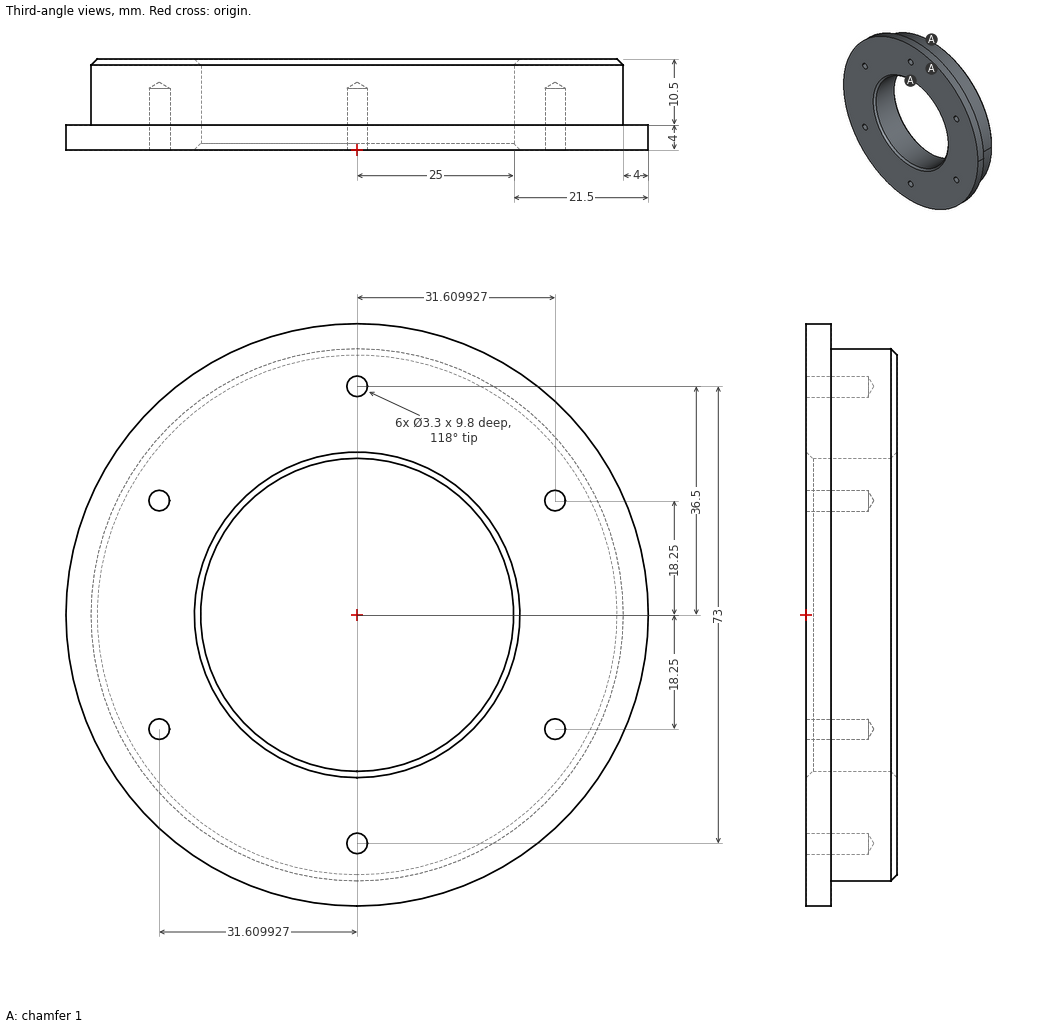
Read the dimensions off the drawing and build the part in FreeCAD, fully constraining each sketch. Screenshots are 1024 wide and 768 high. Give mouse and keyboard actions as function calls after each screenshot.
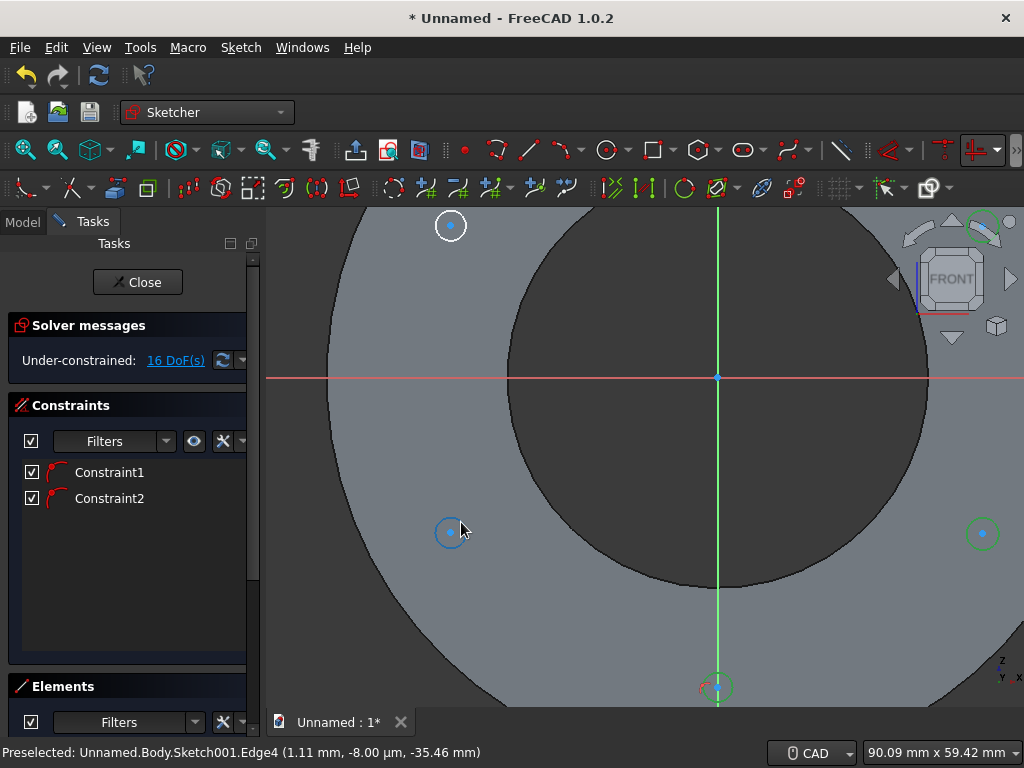
click(462, 522)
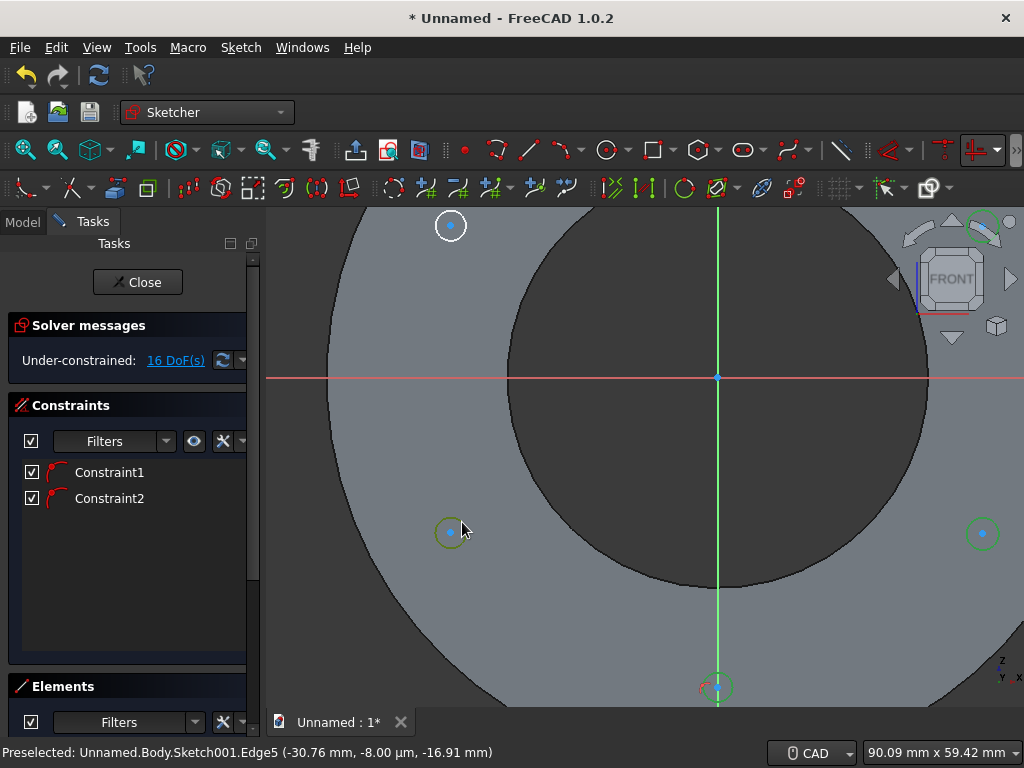
click(440, 236)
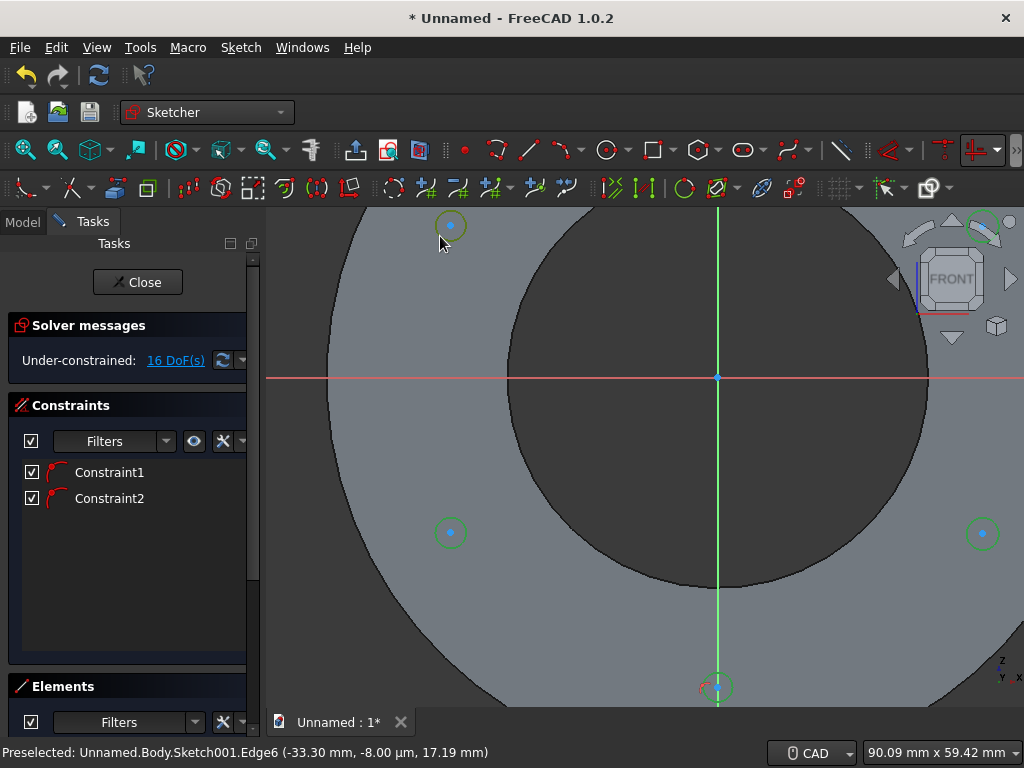
key(e)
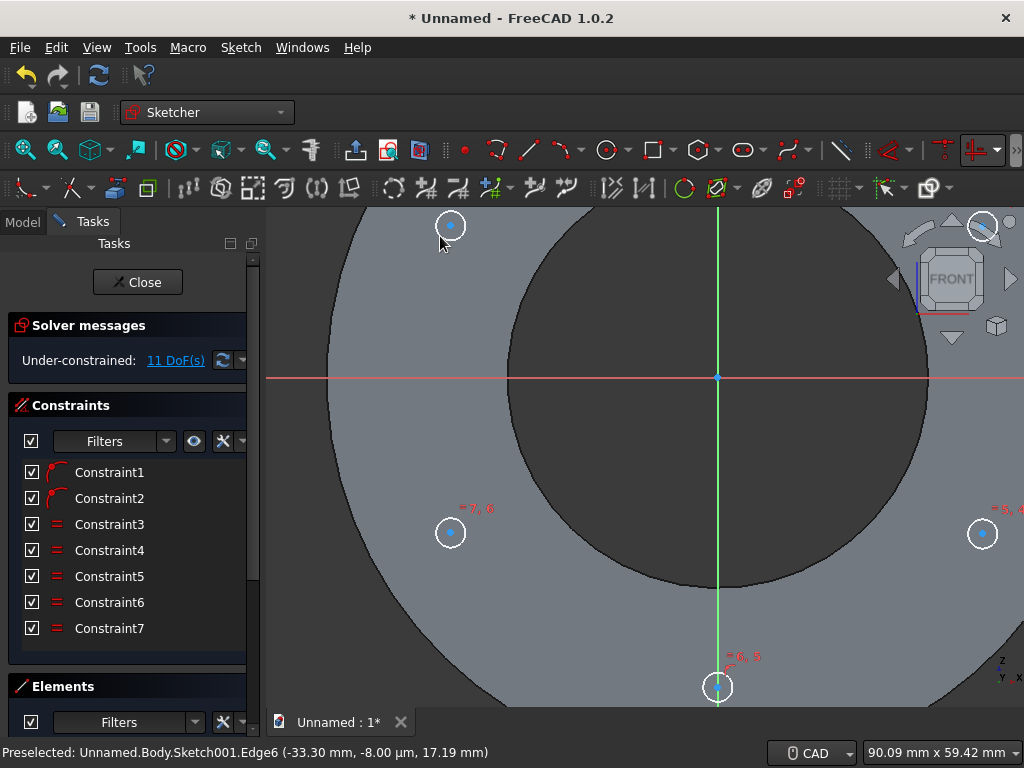
scroll(461, 522, down, 4)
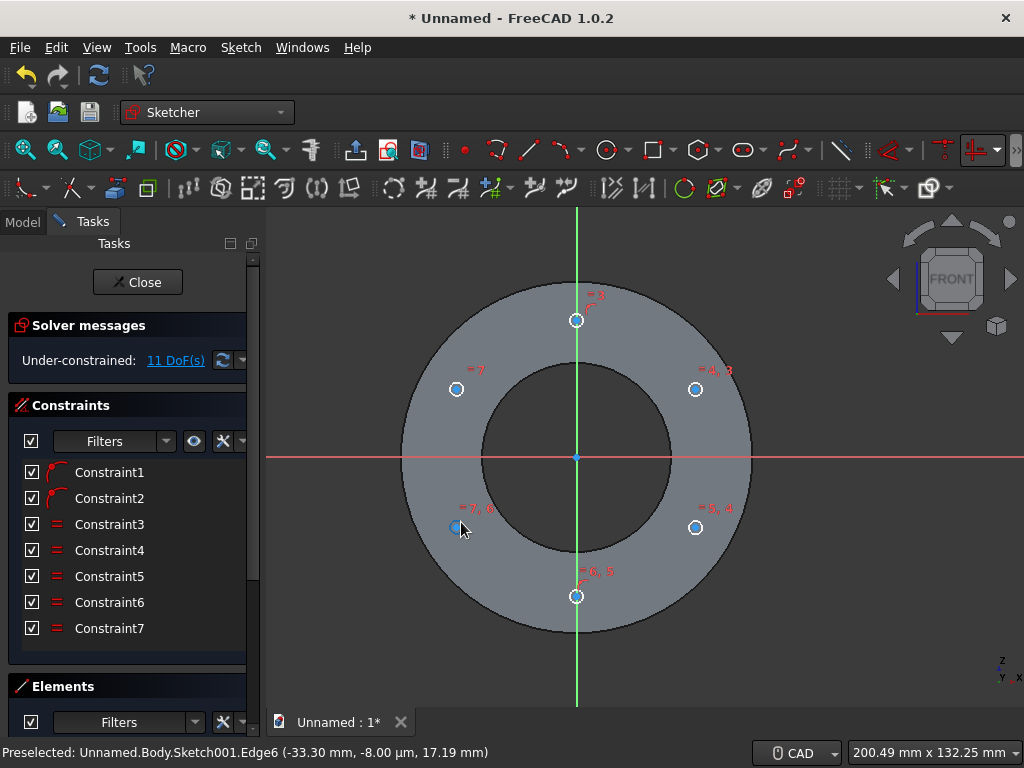
click(696, 389)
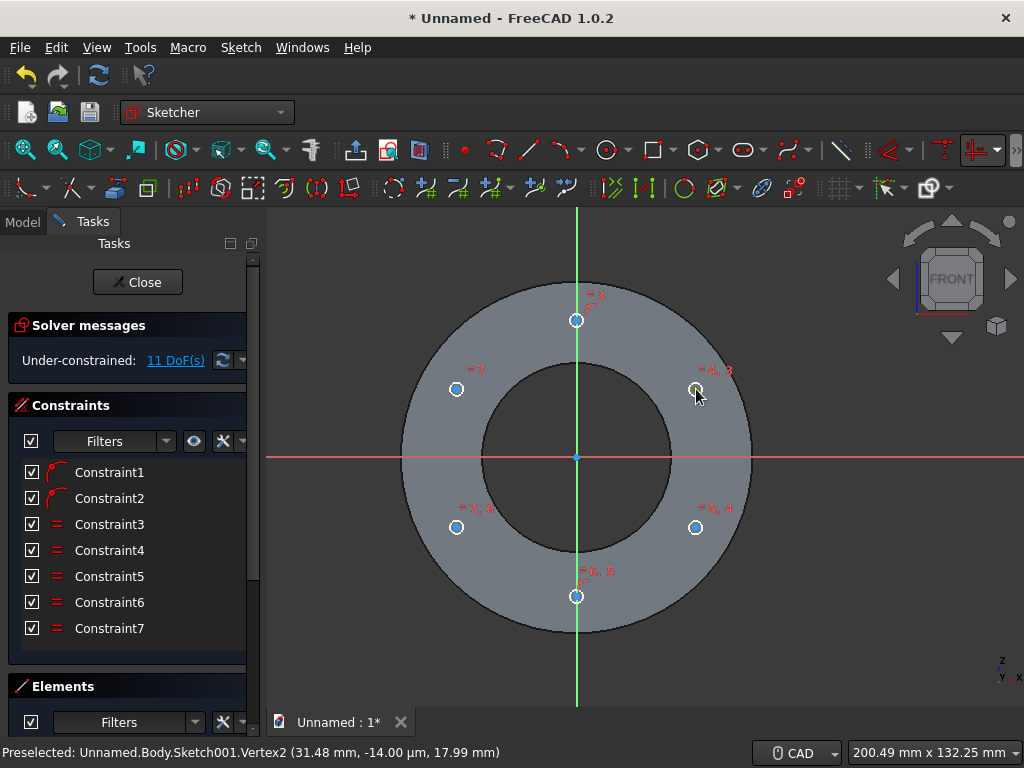
click(696, 528)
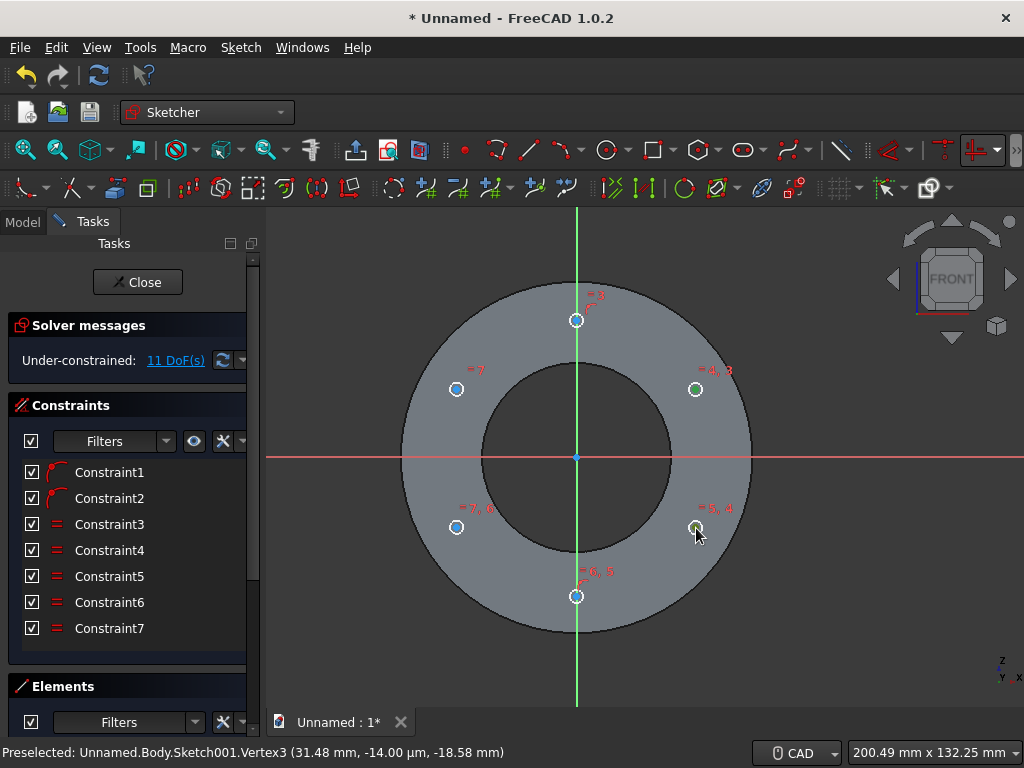
key(v)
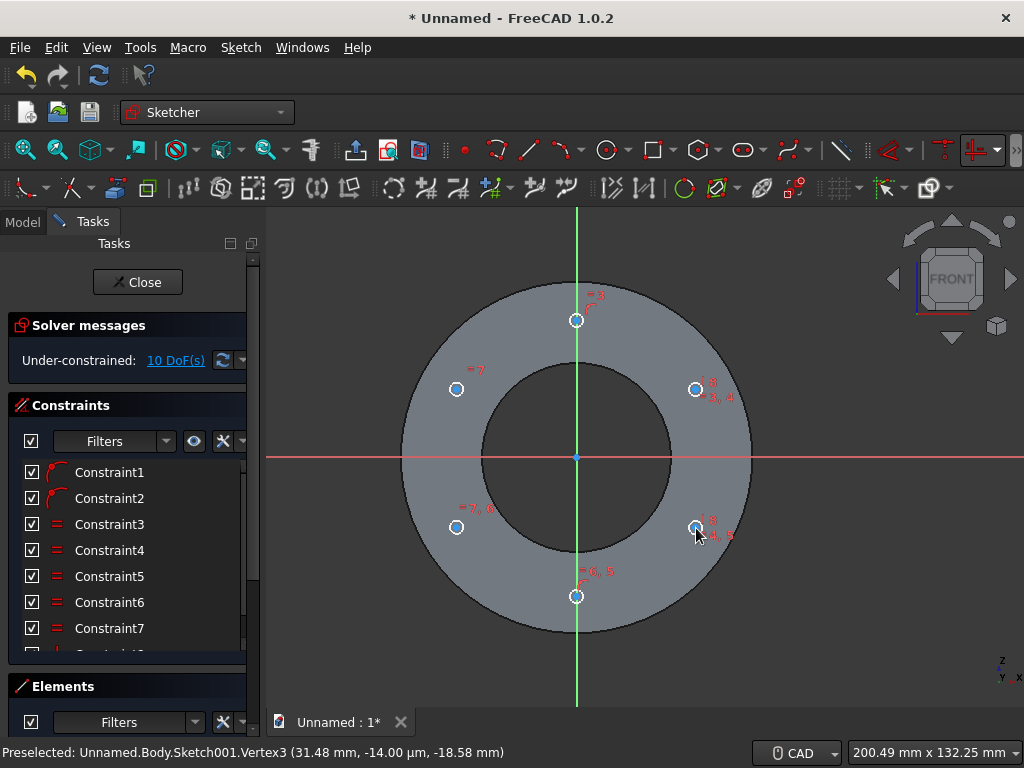
click(696, 528)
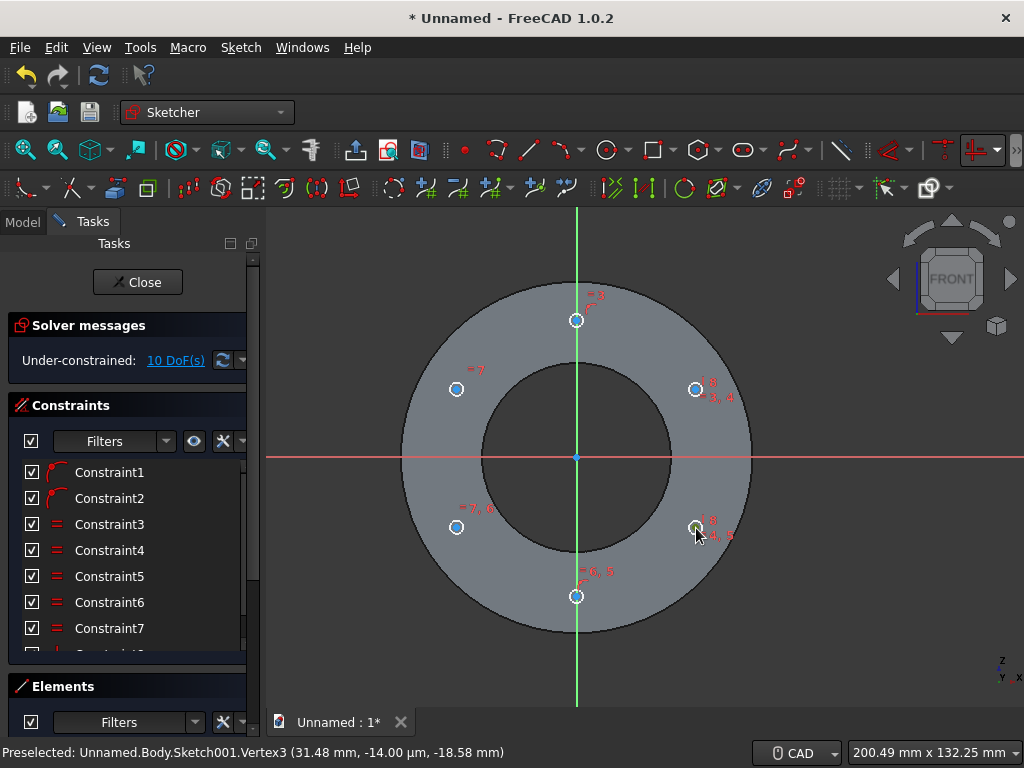
click(457, 527)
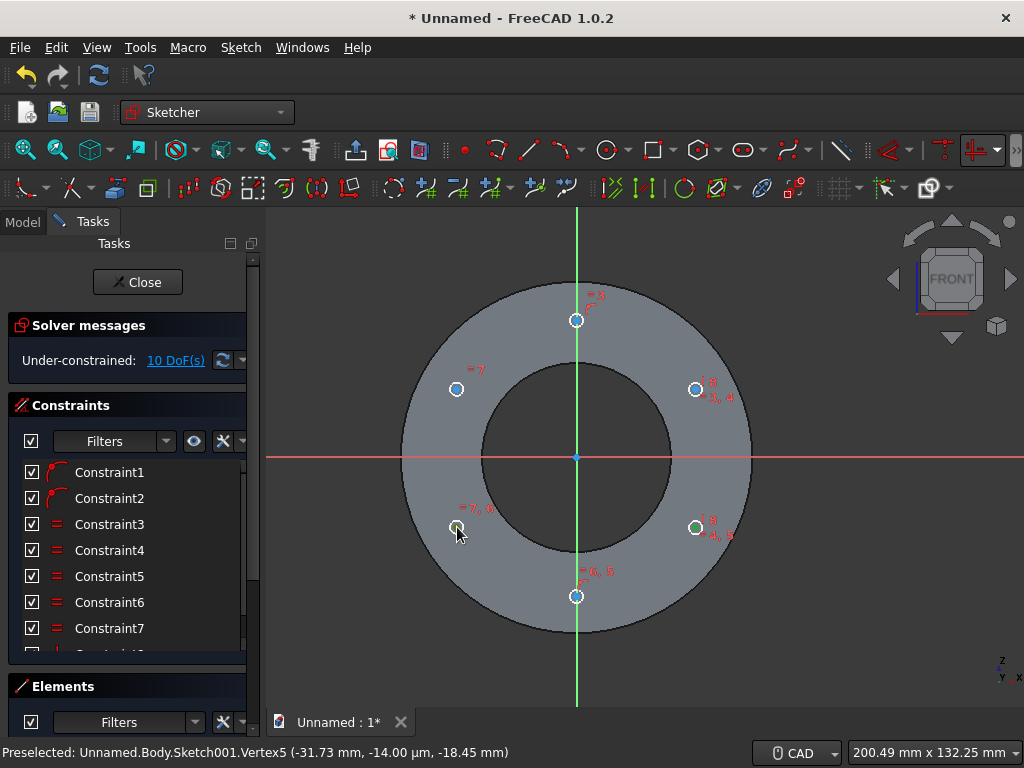
key(h)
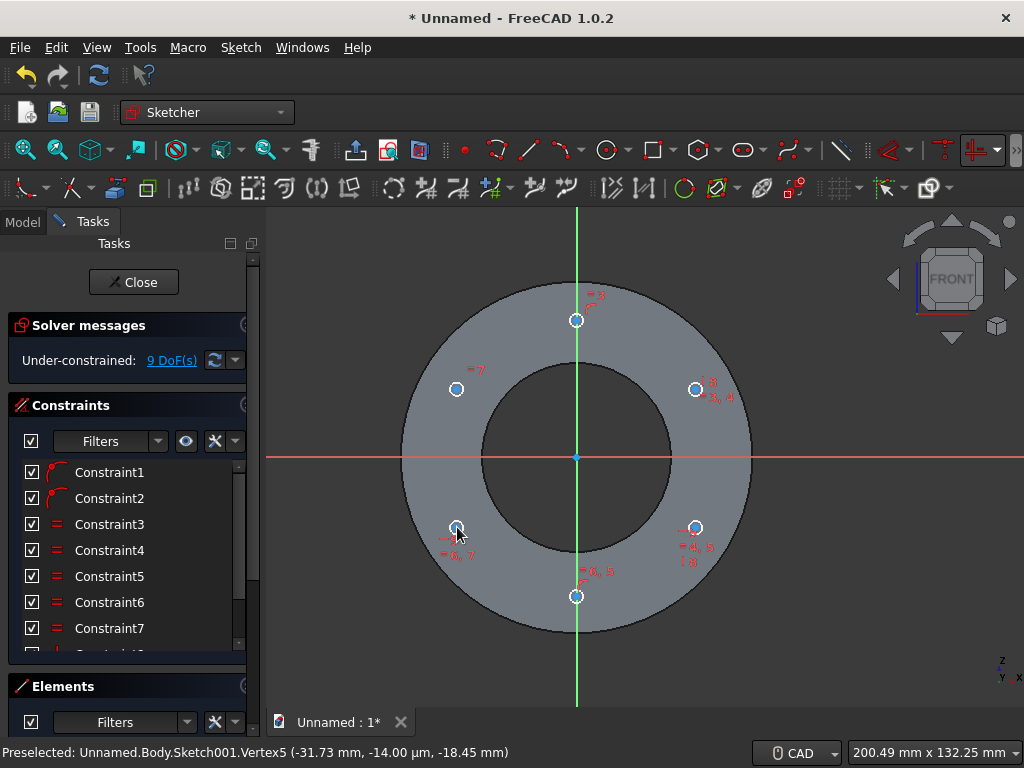
click(457, 528)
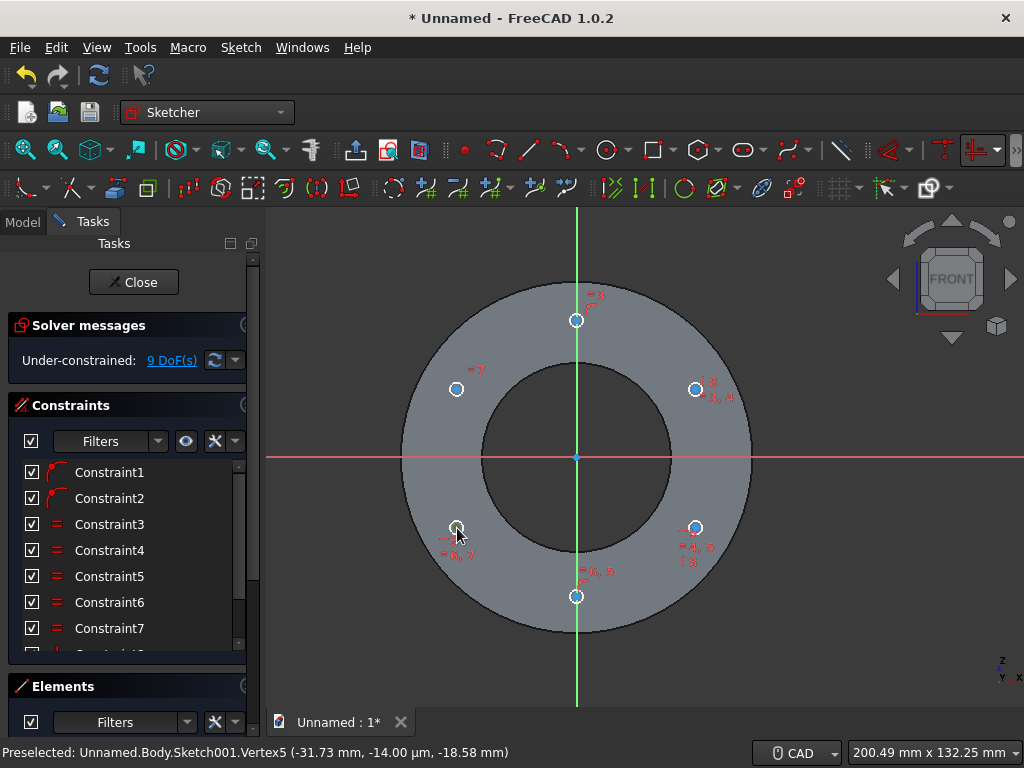
click(457, 389)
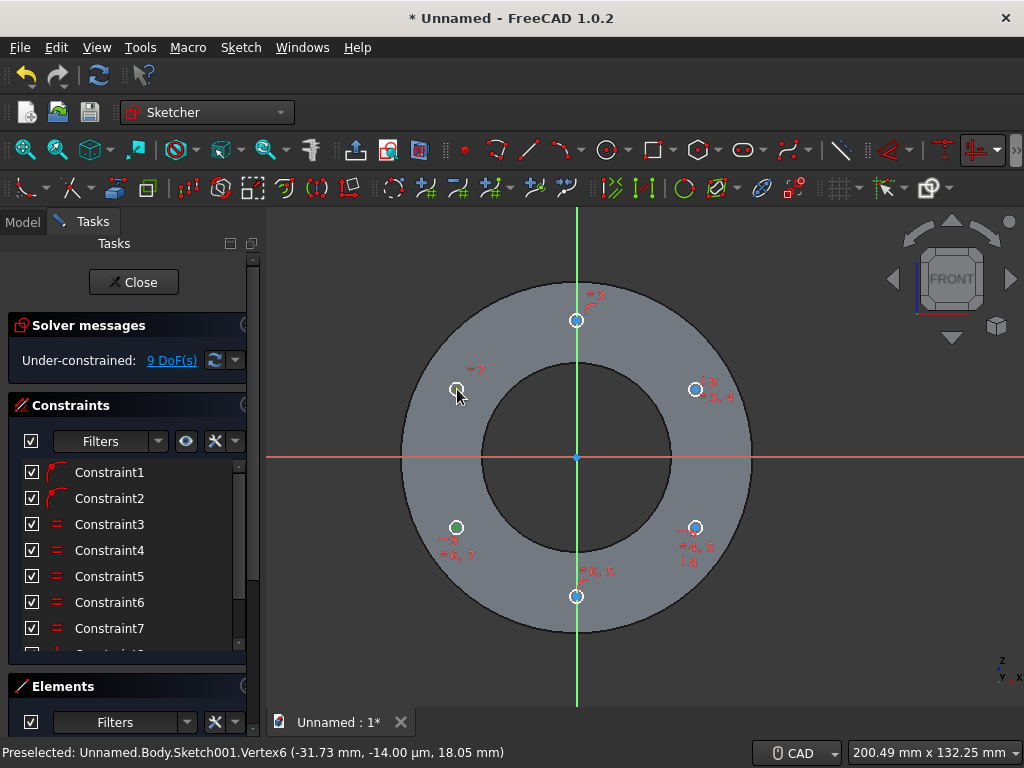
key(v)